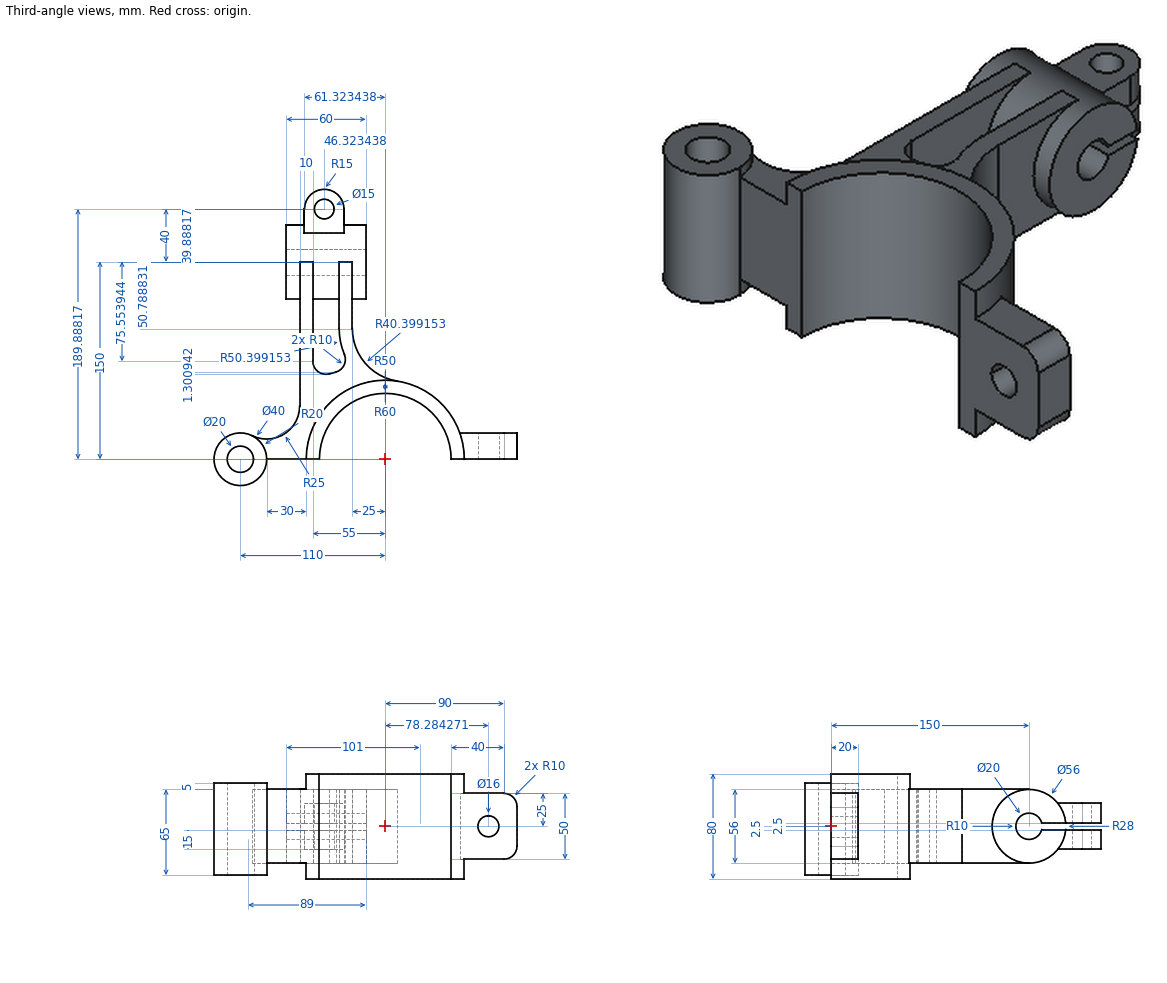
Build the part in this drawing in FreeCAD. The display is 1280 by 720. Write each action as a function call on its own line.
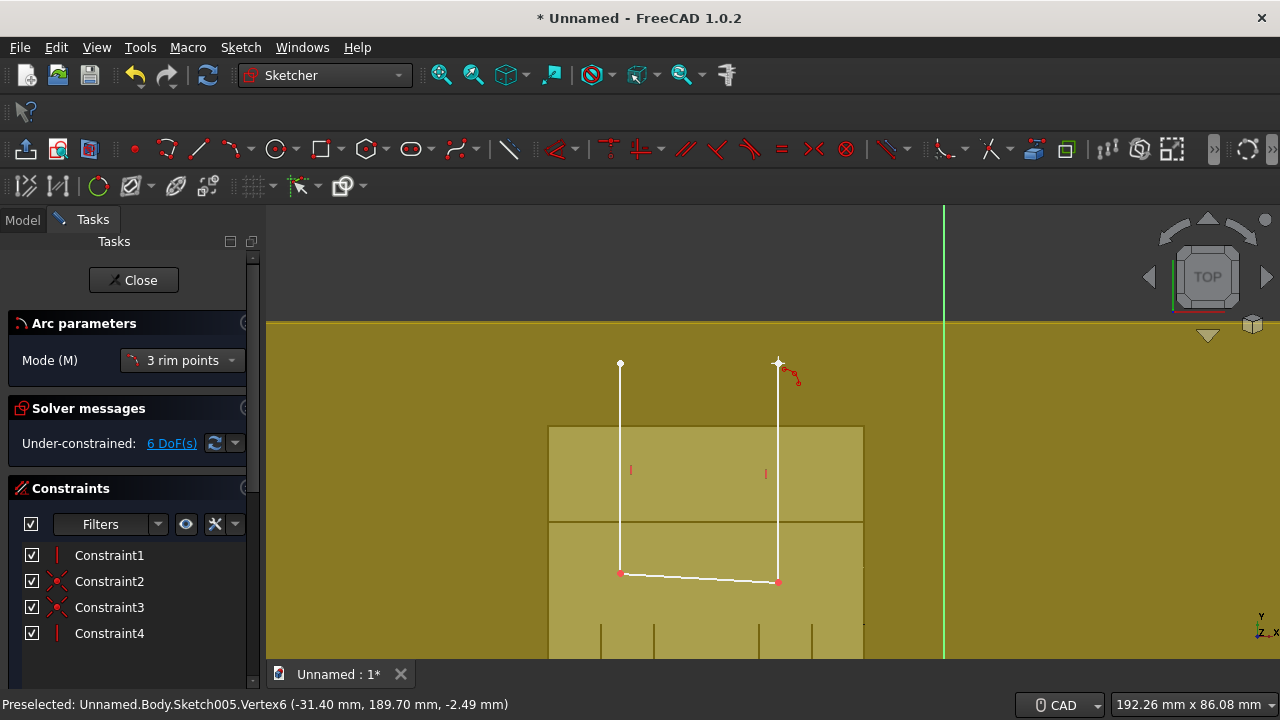
click(778, 364)
click(620, 364)
click(699, 284)
key(Escape)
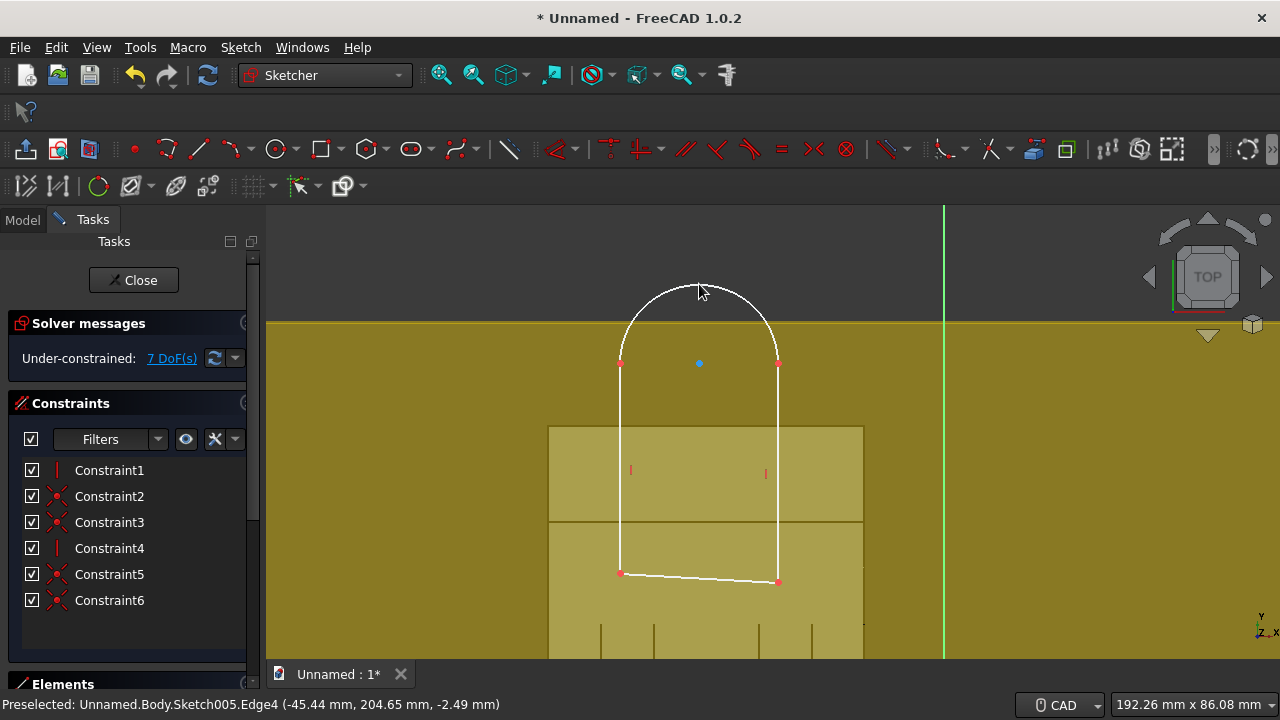
click(620, 427)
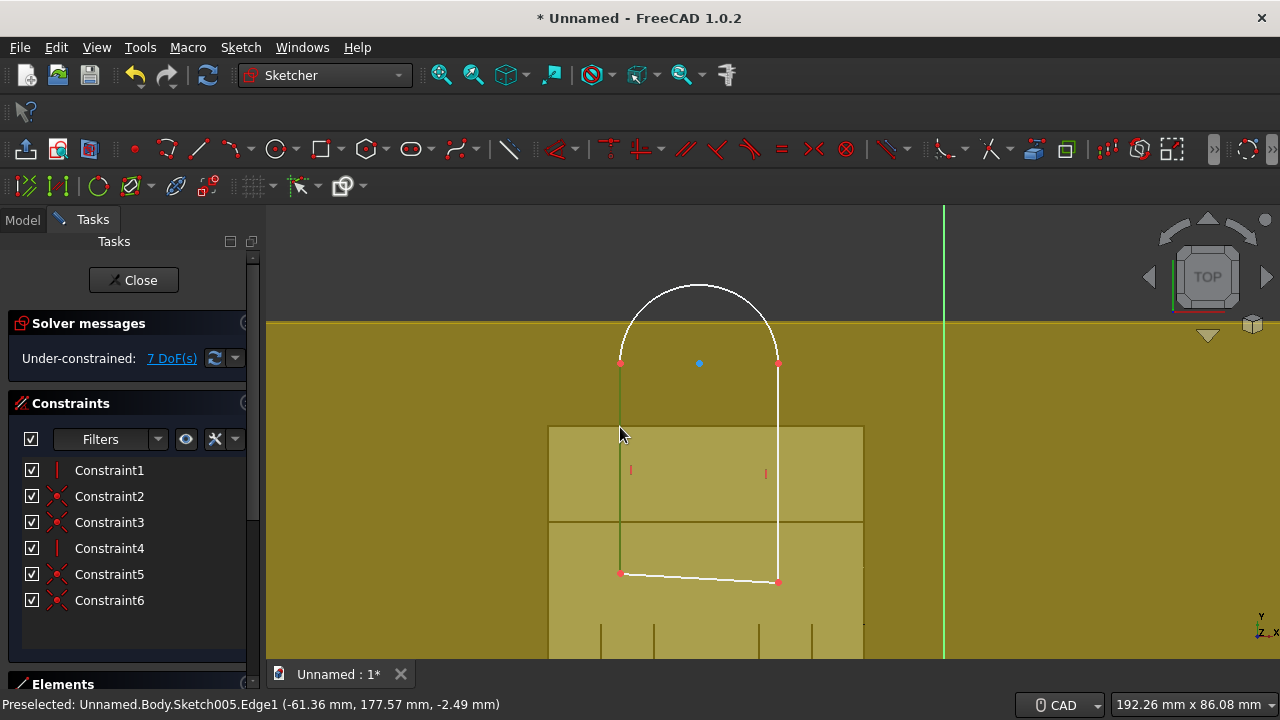
click(745, 300)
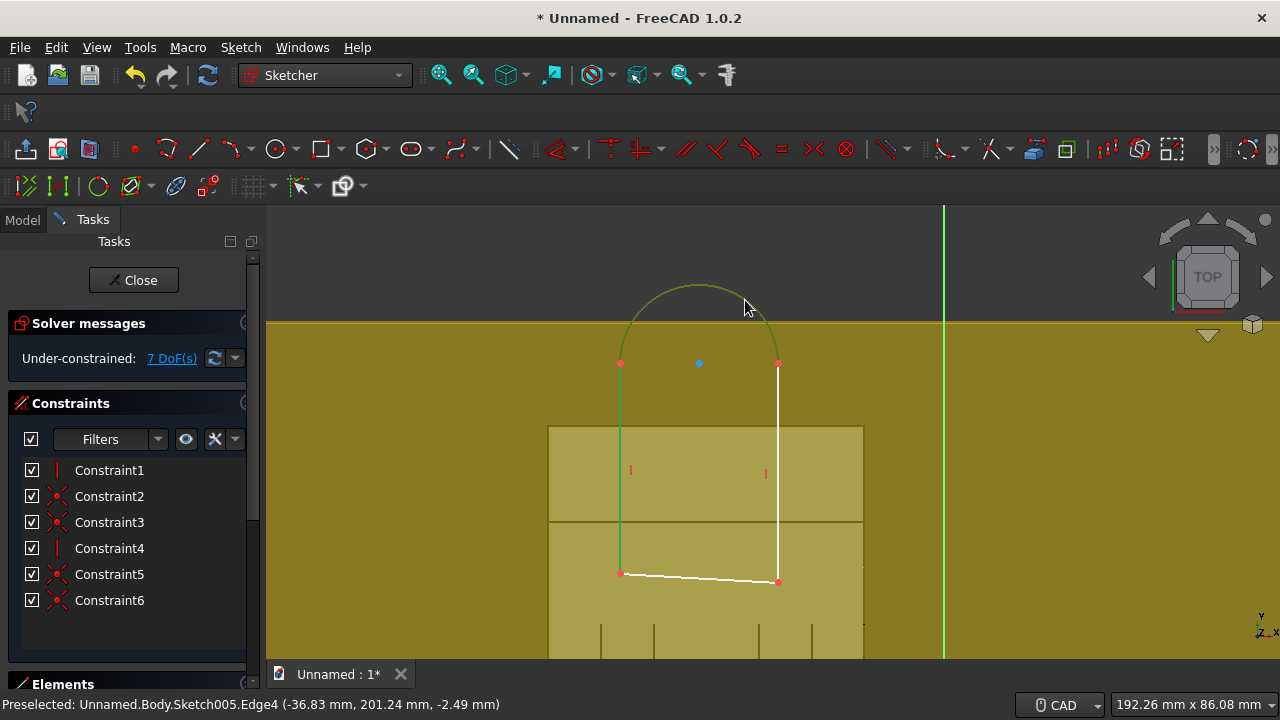
key(t)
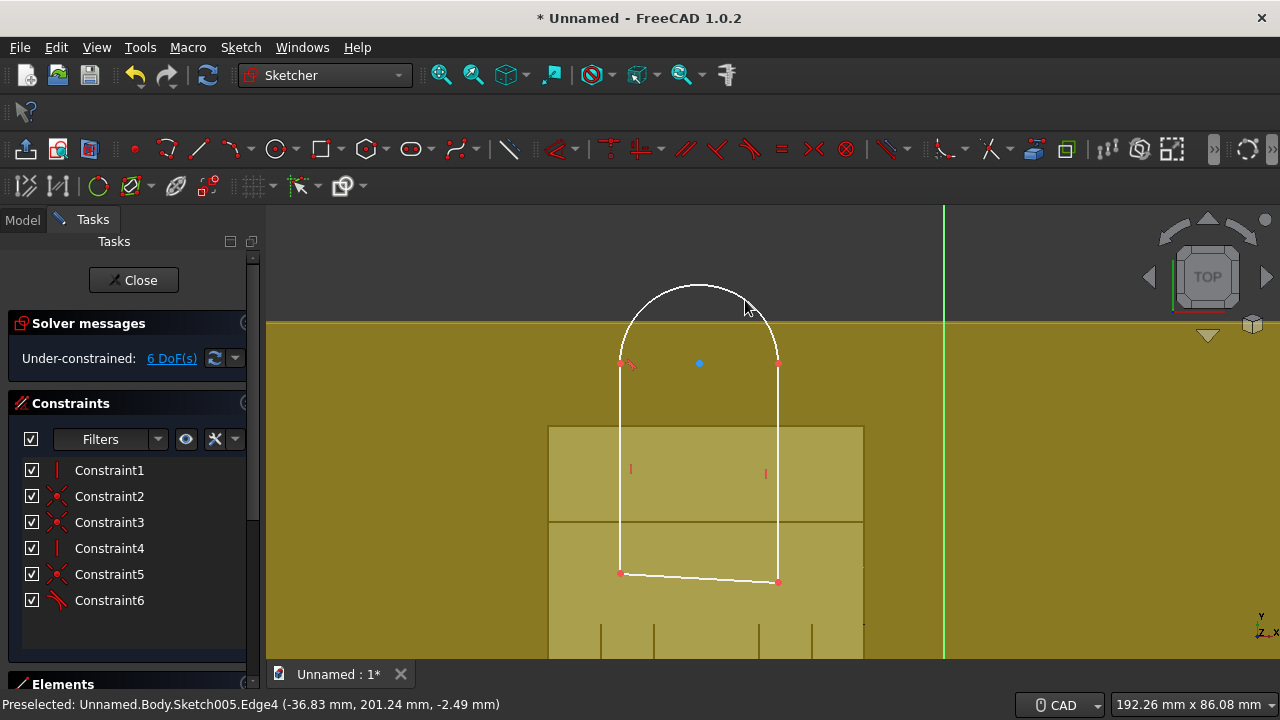
click(778, 517)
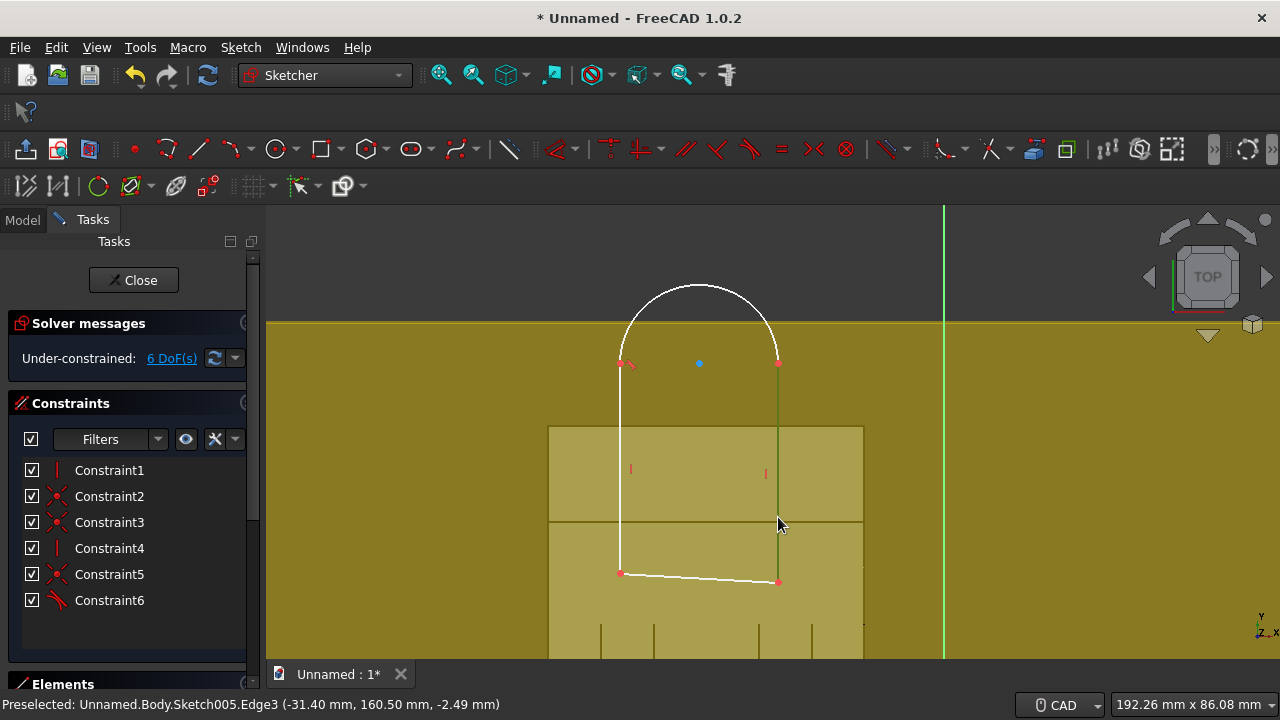
click(745, 300)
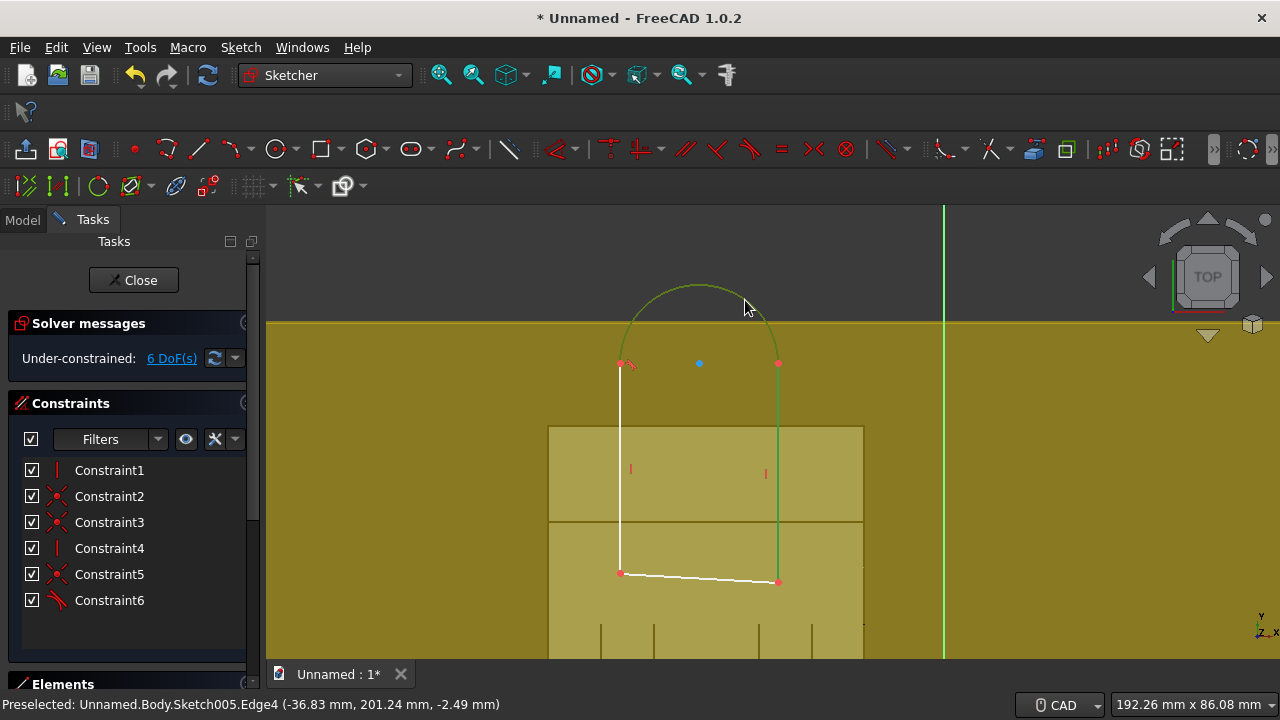
click(750, 150)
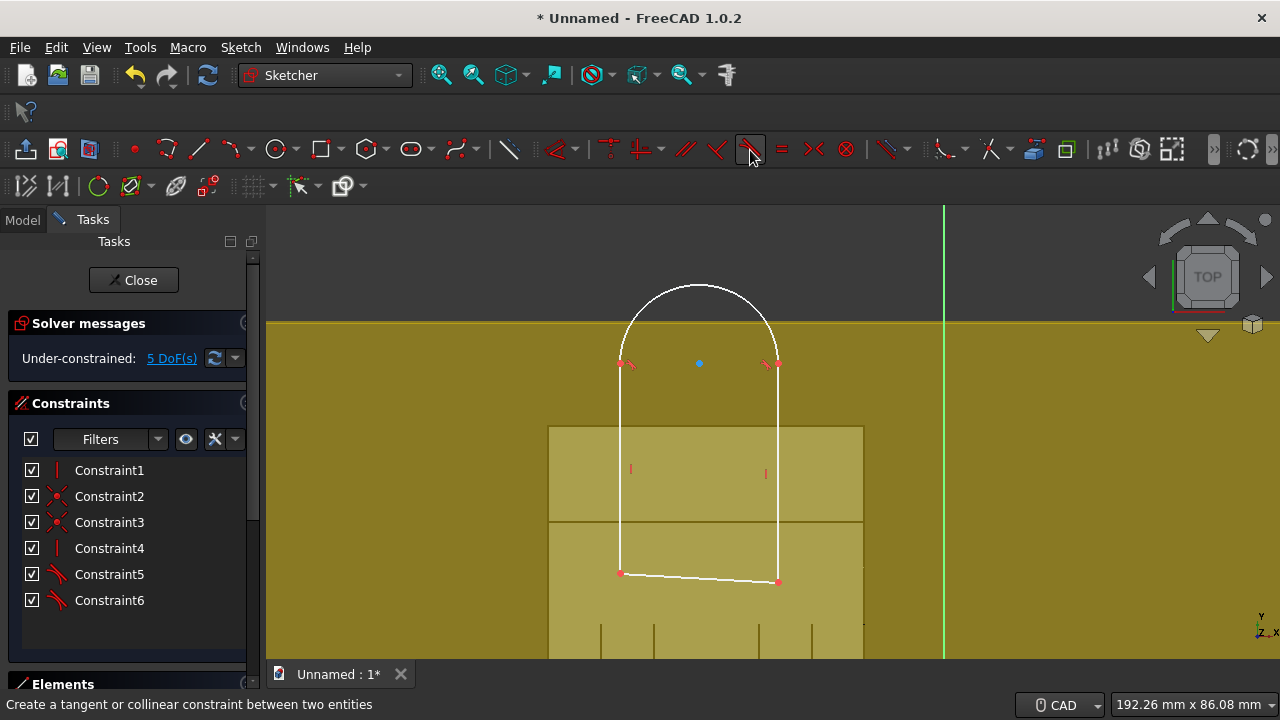
key(d)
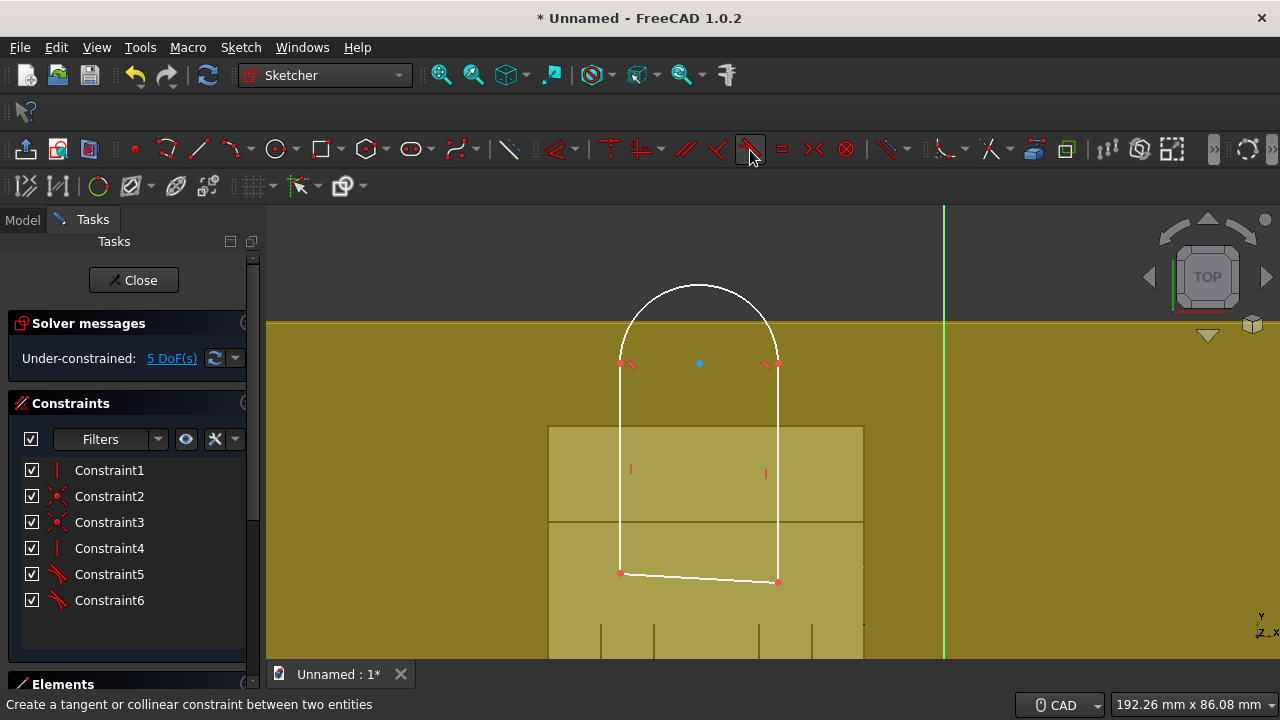
click(745, 300)
click(764, 274)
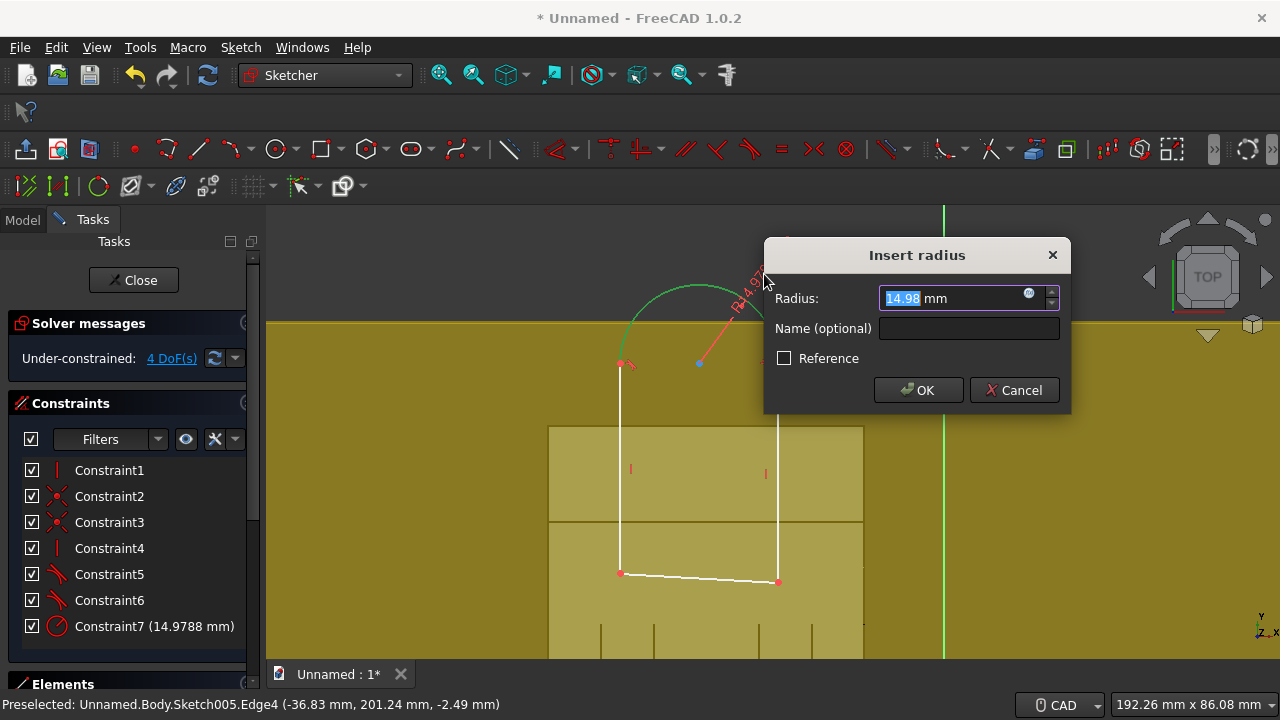
text(15)
key(Return)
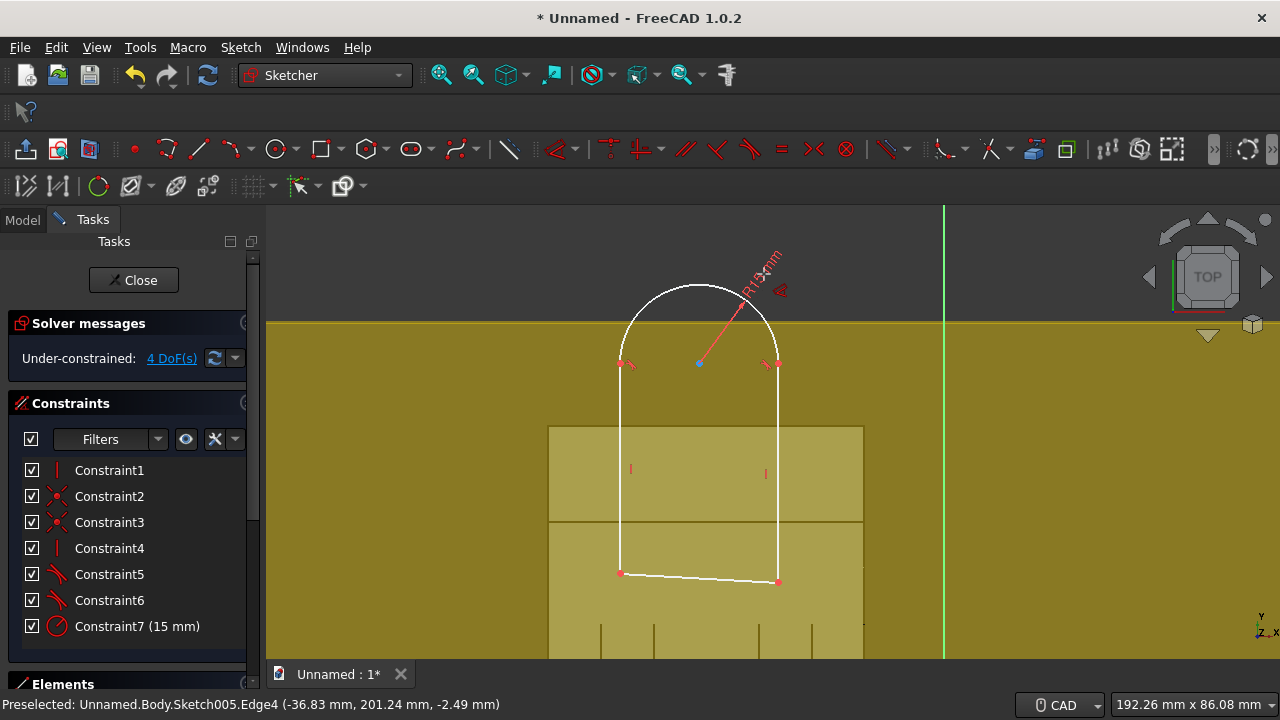
click(778, 517)
click(812, 473)